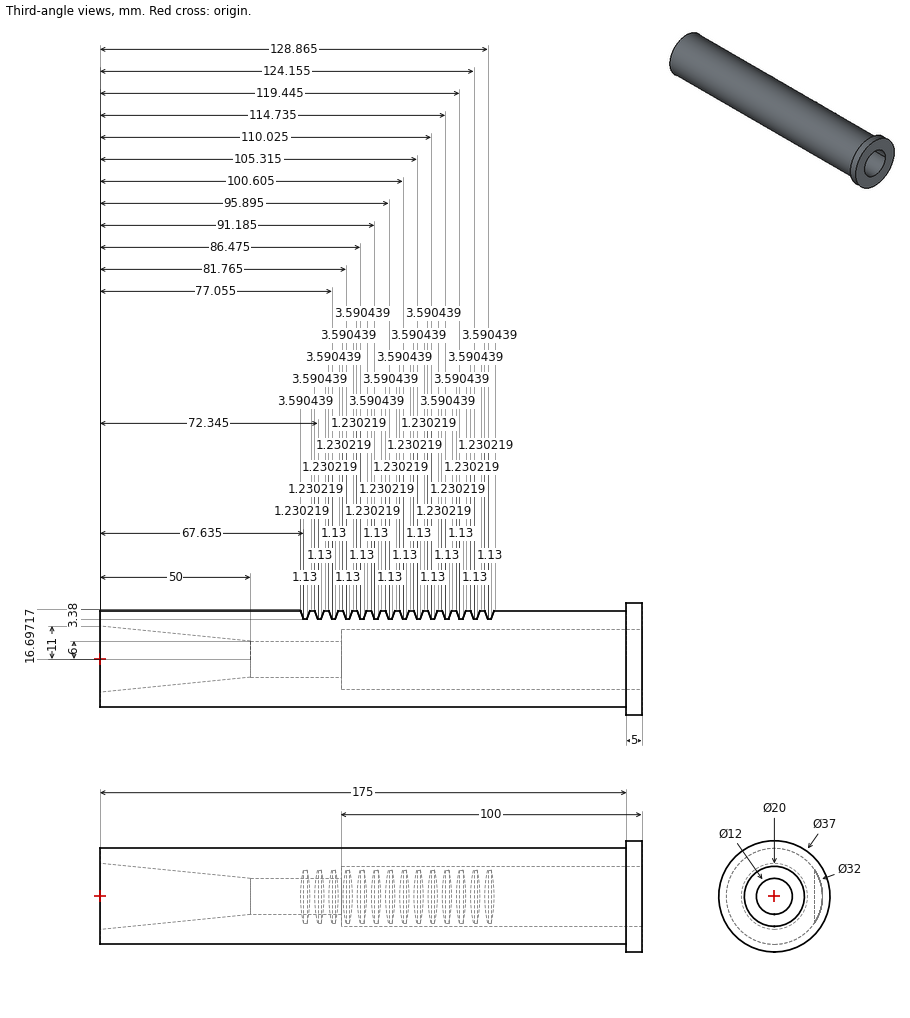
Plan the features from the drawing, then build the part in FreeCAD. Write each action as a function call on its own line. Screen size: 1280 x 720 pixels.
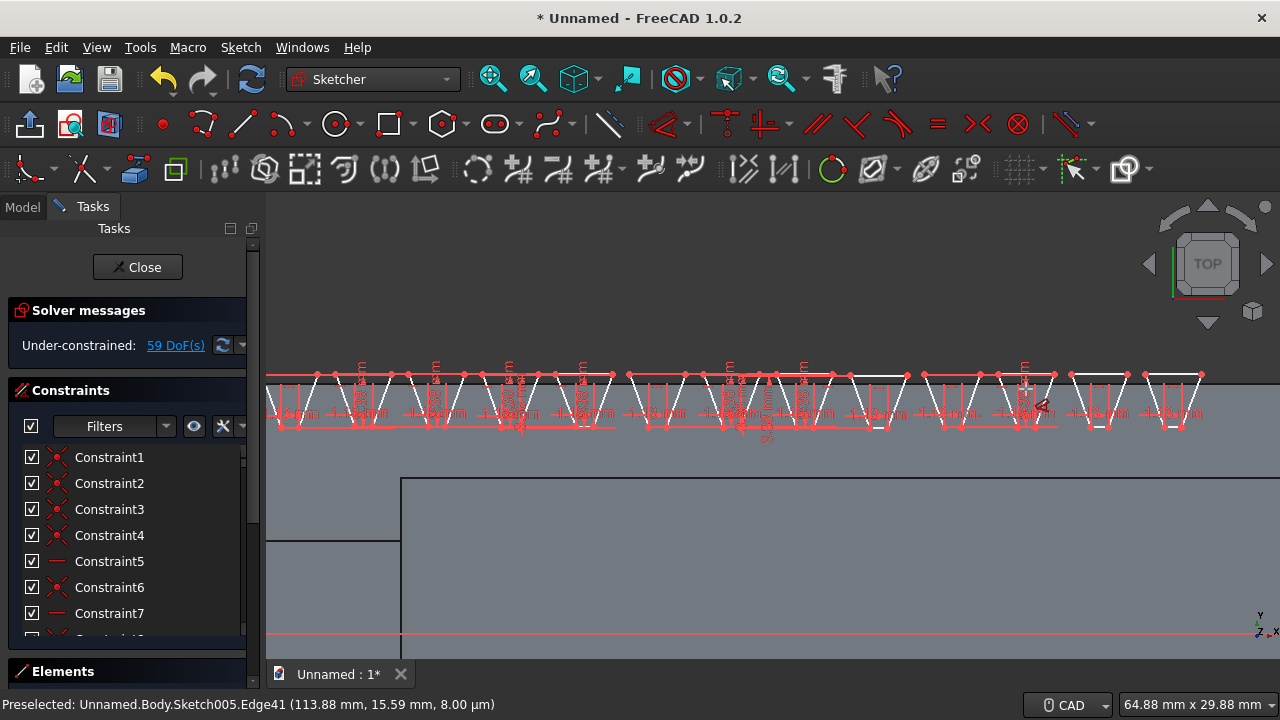
click(1004, 390)
click(1100, 389)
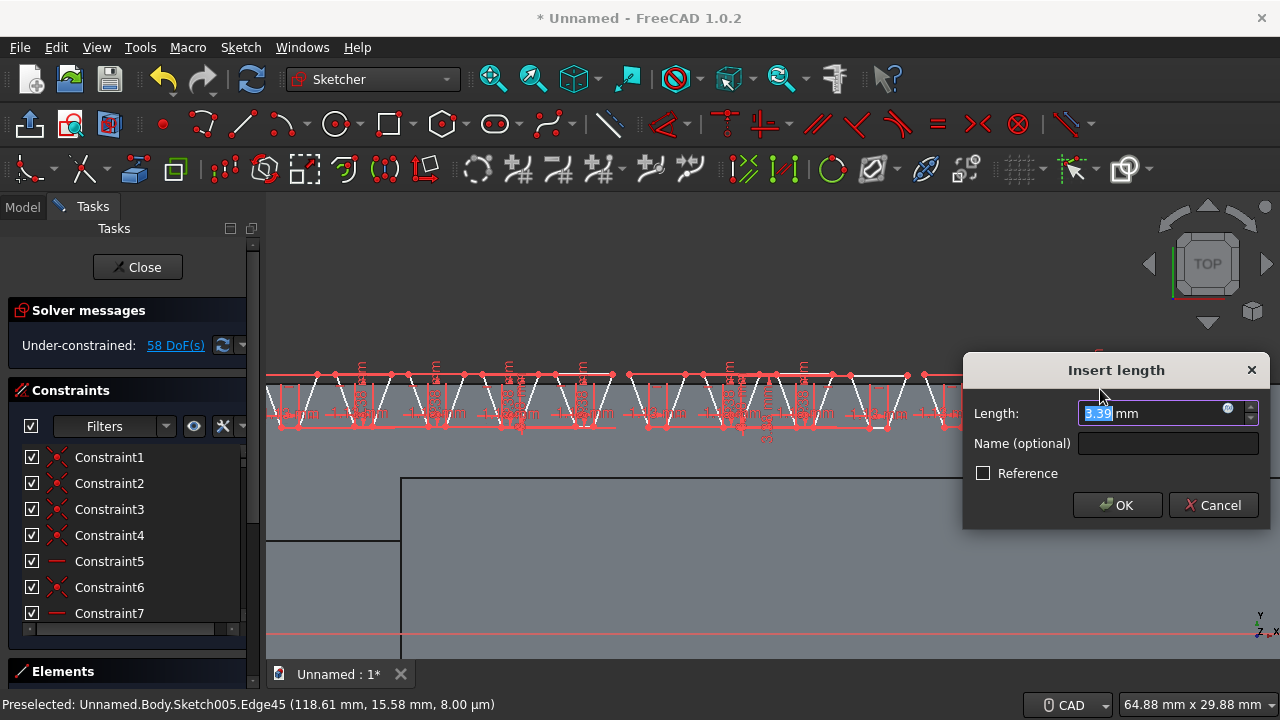
text(3.38)
key(Return)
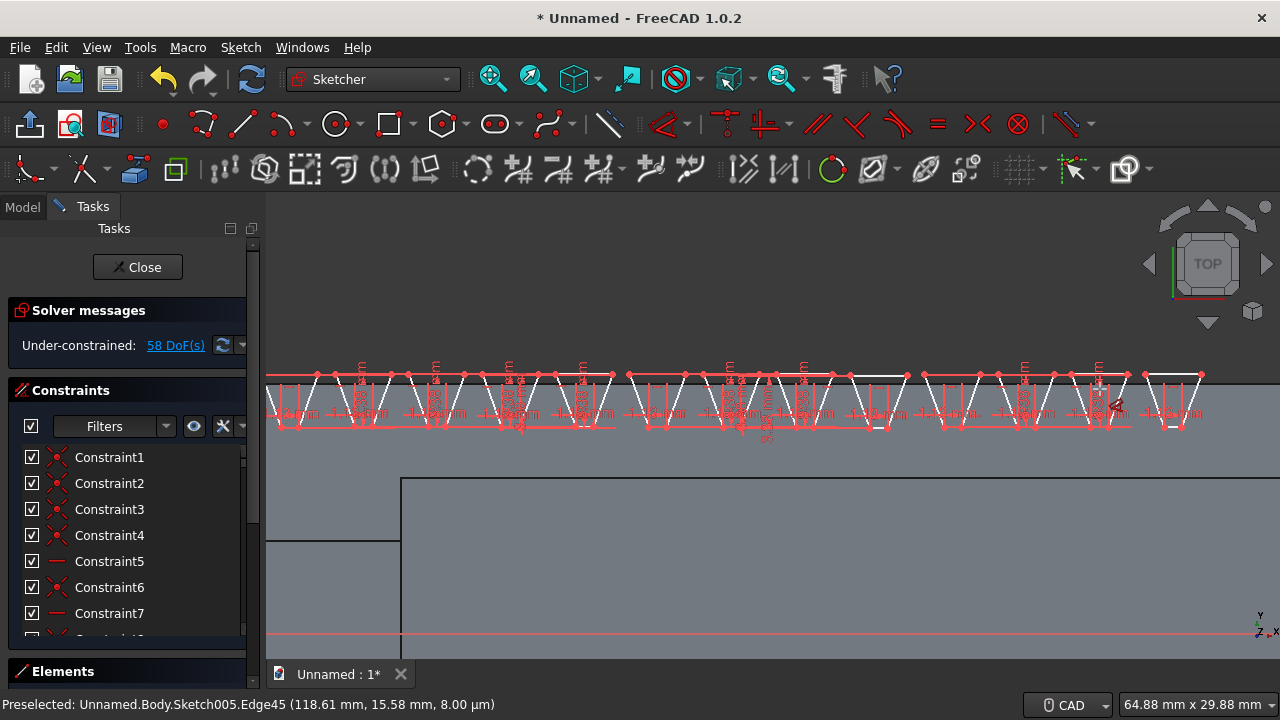
click(1078, 390)
click(1038, 401)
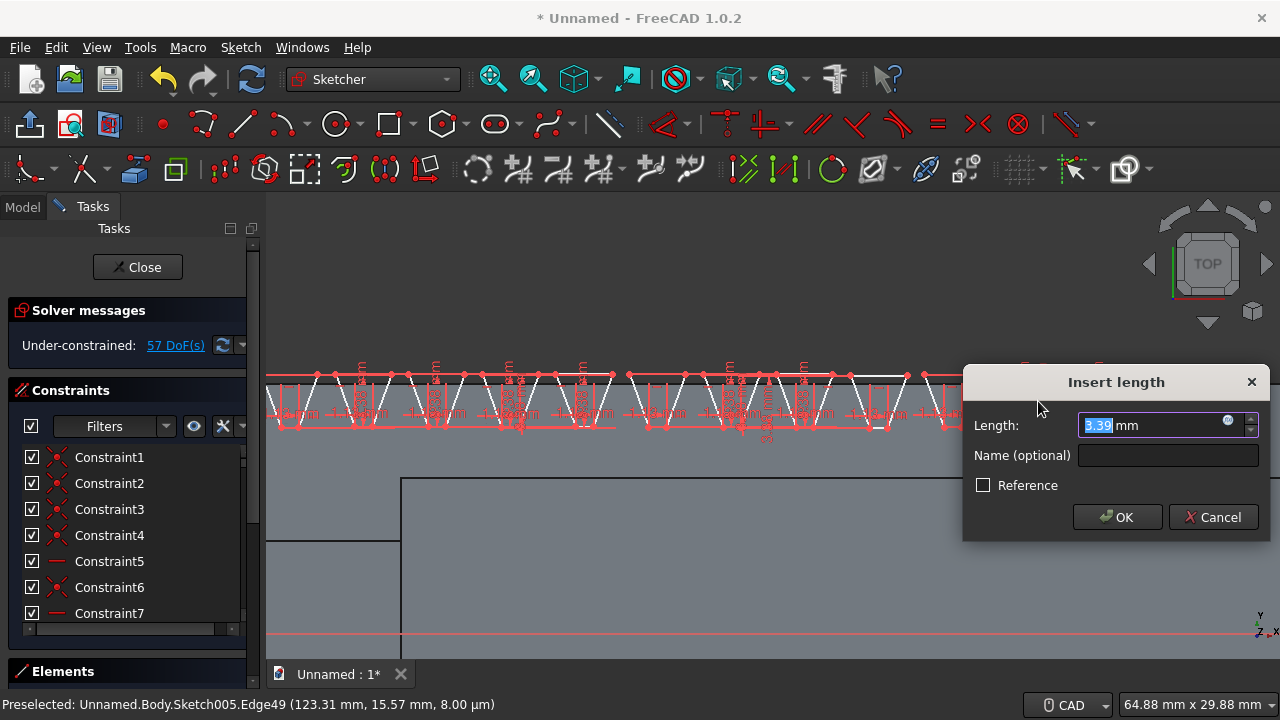
text(3.38)
key(Return)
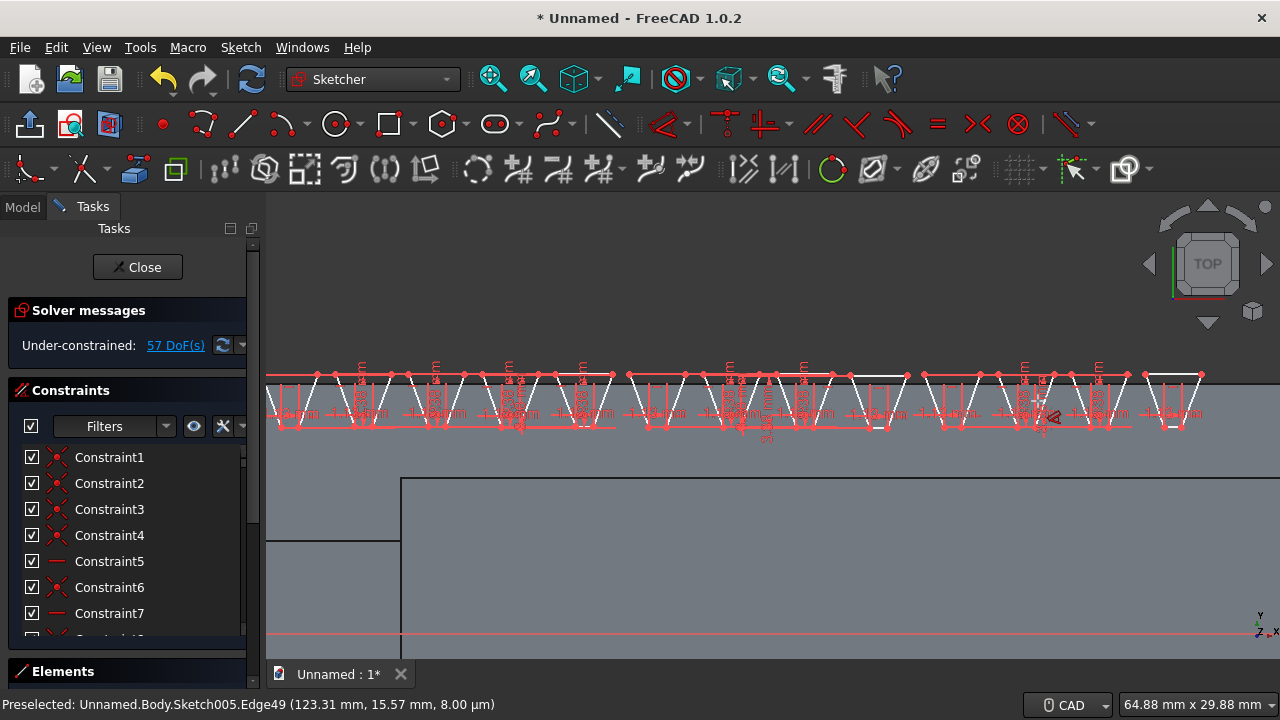
scroll(932, 392, down, 6)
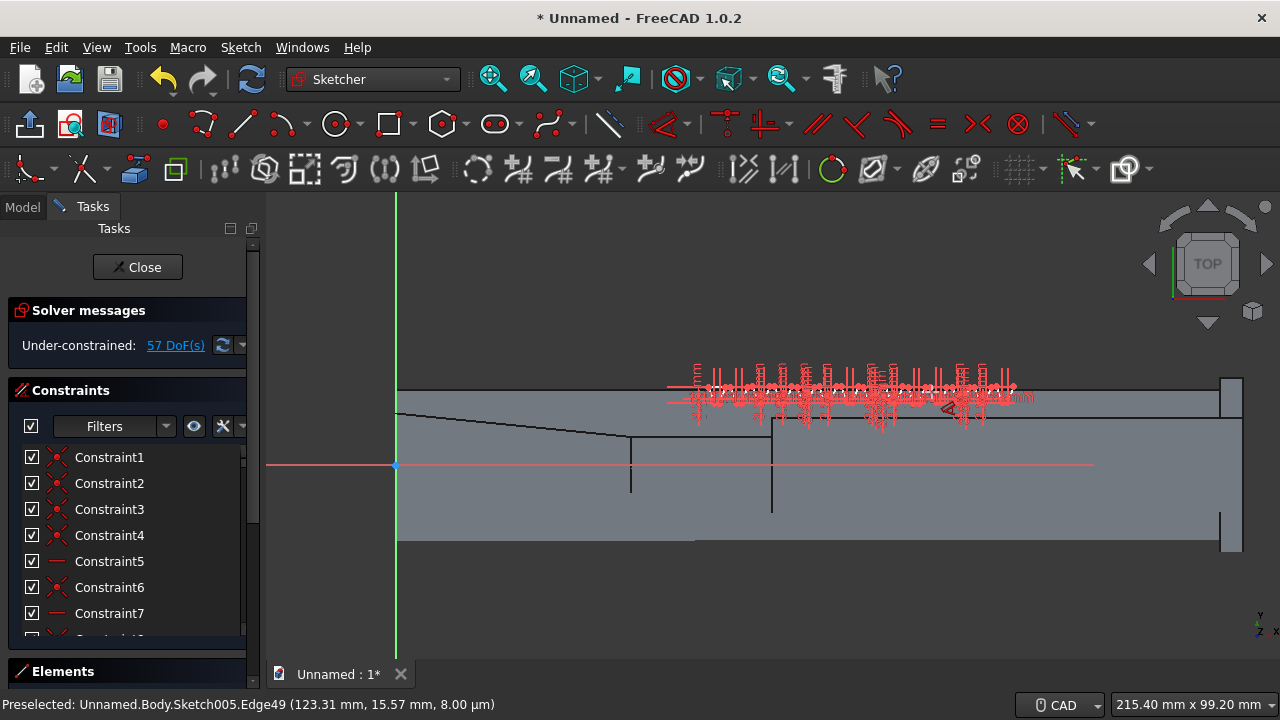
scroll(999, 392, up, 6)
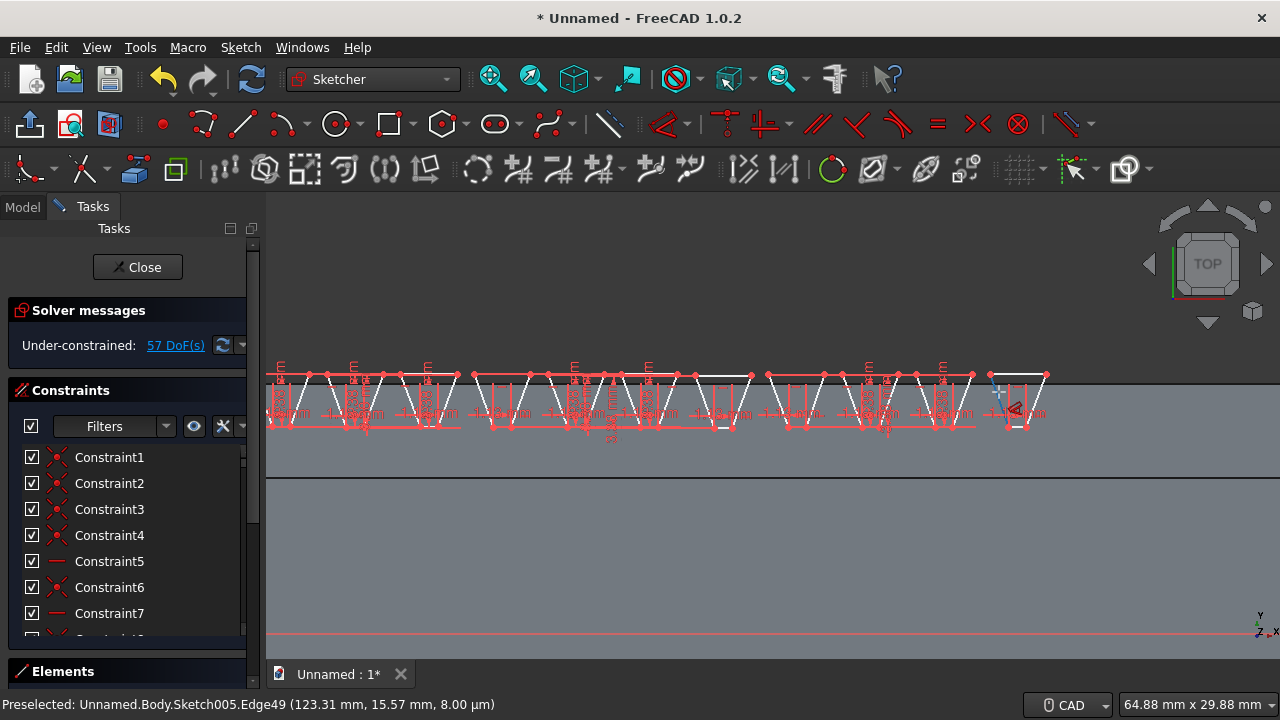
click(996, 390)
click(1067, 389)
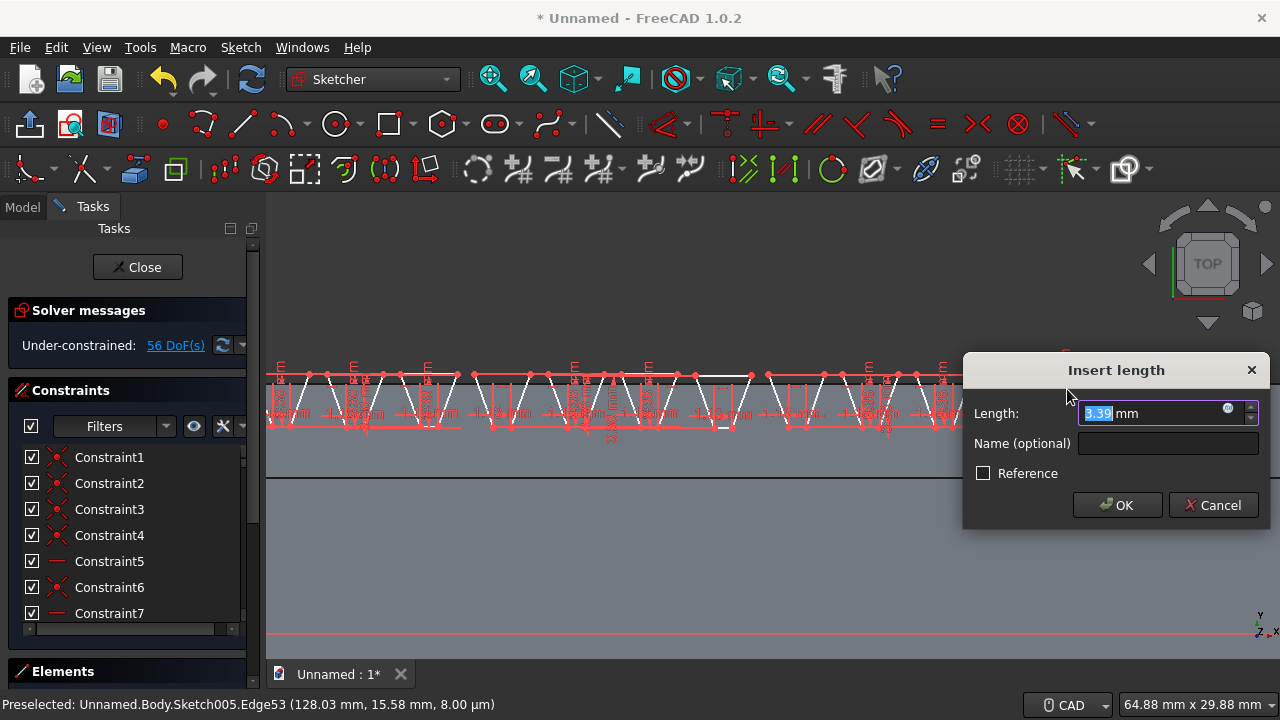
text(3.38)
key(Return)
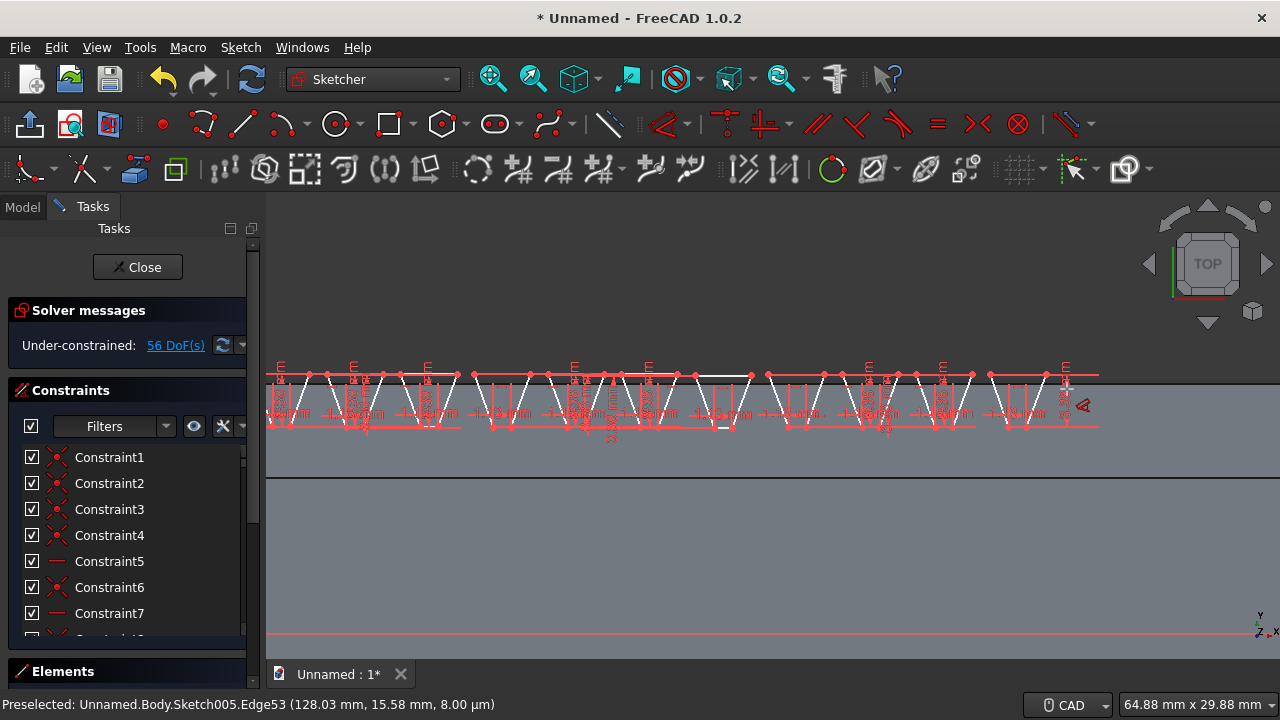
scroll(999, 392, down, 6)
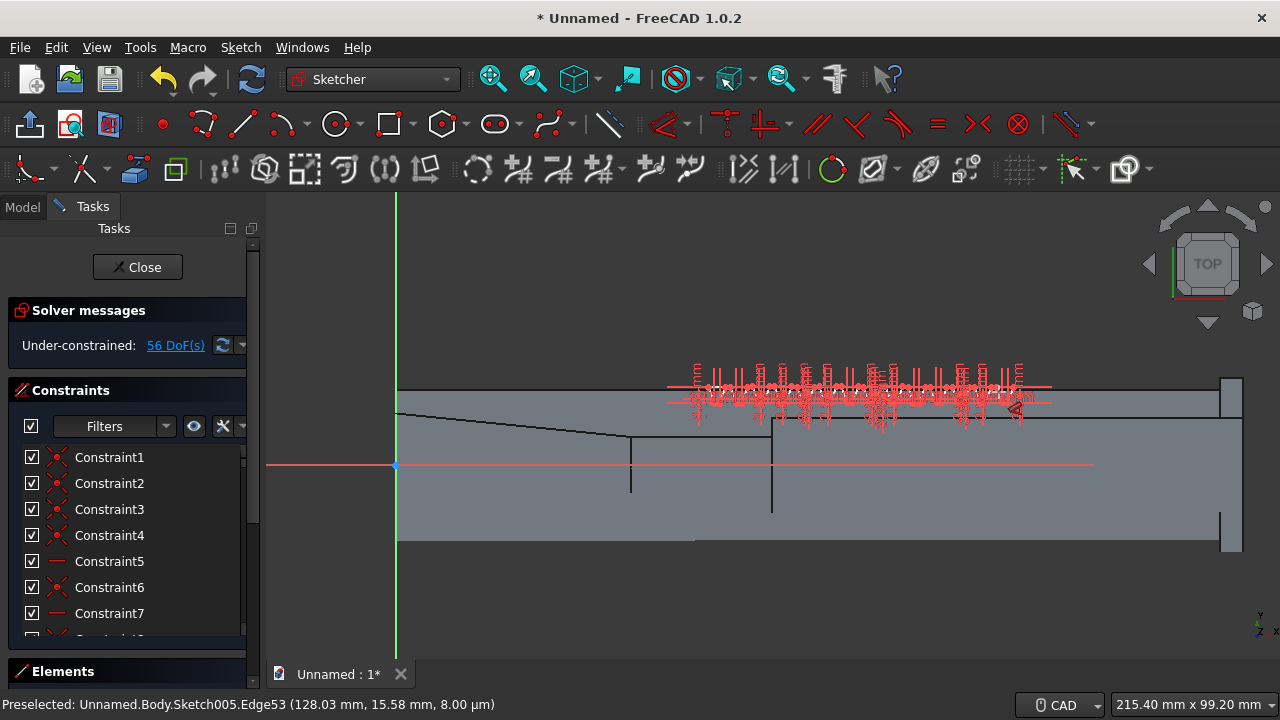
scroll(714, 403, up, 5)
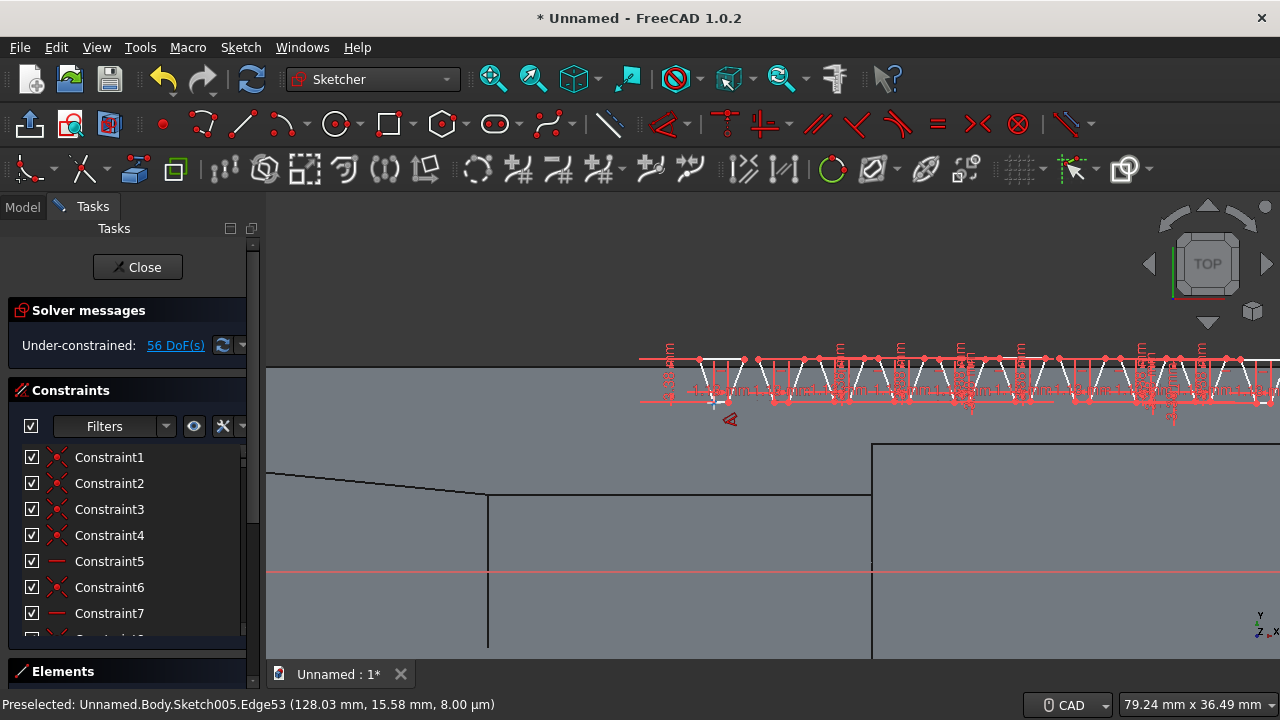
click(714, 402)
click(504, 606)